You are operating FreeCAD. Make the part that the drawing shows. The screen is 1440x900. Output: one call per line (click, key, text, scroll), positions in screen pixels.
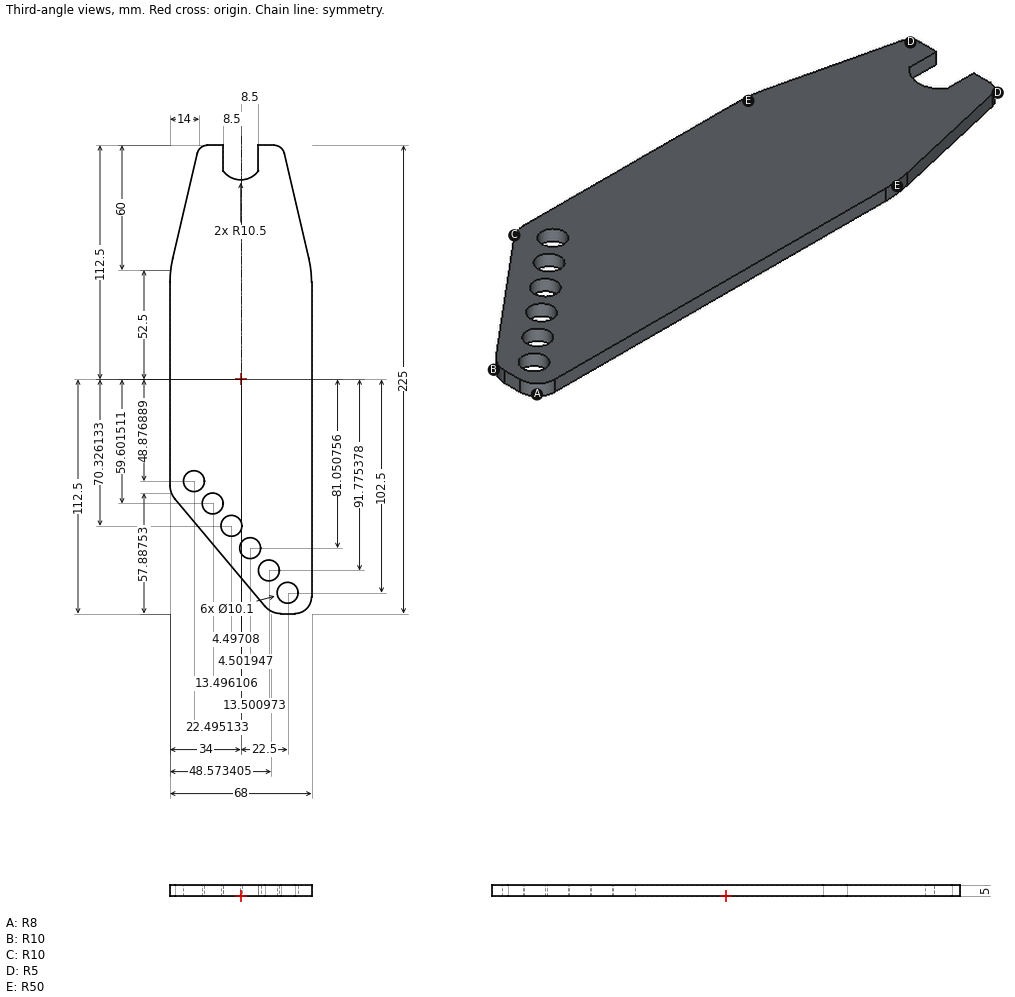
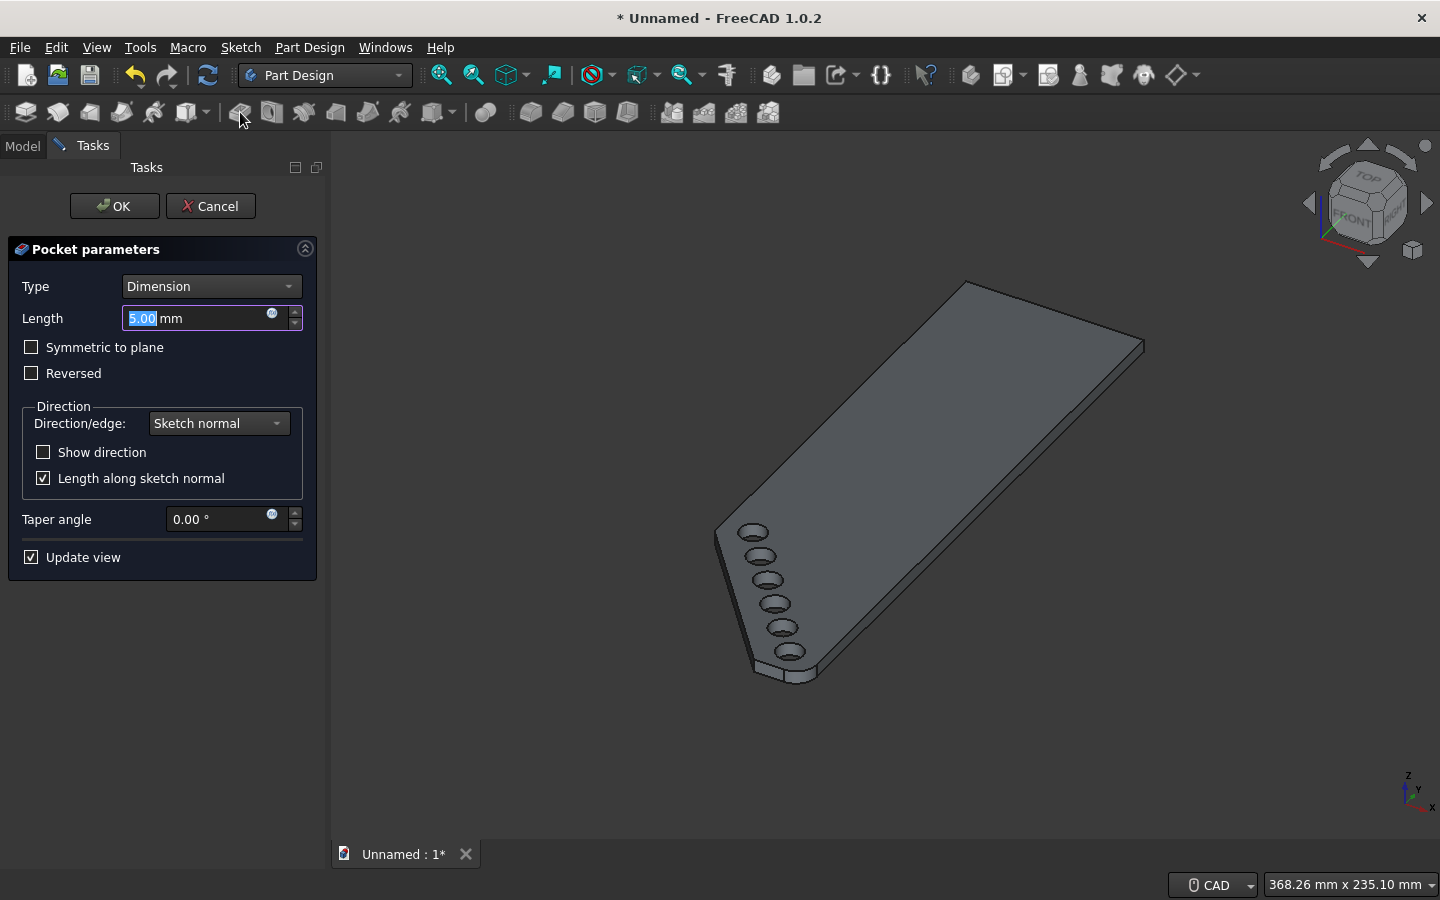
click(212, 286)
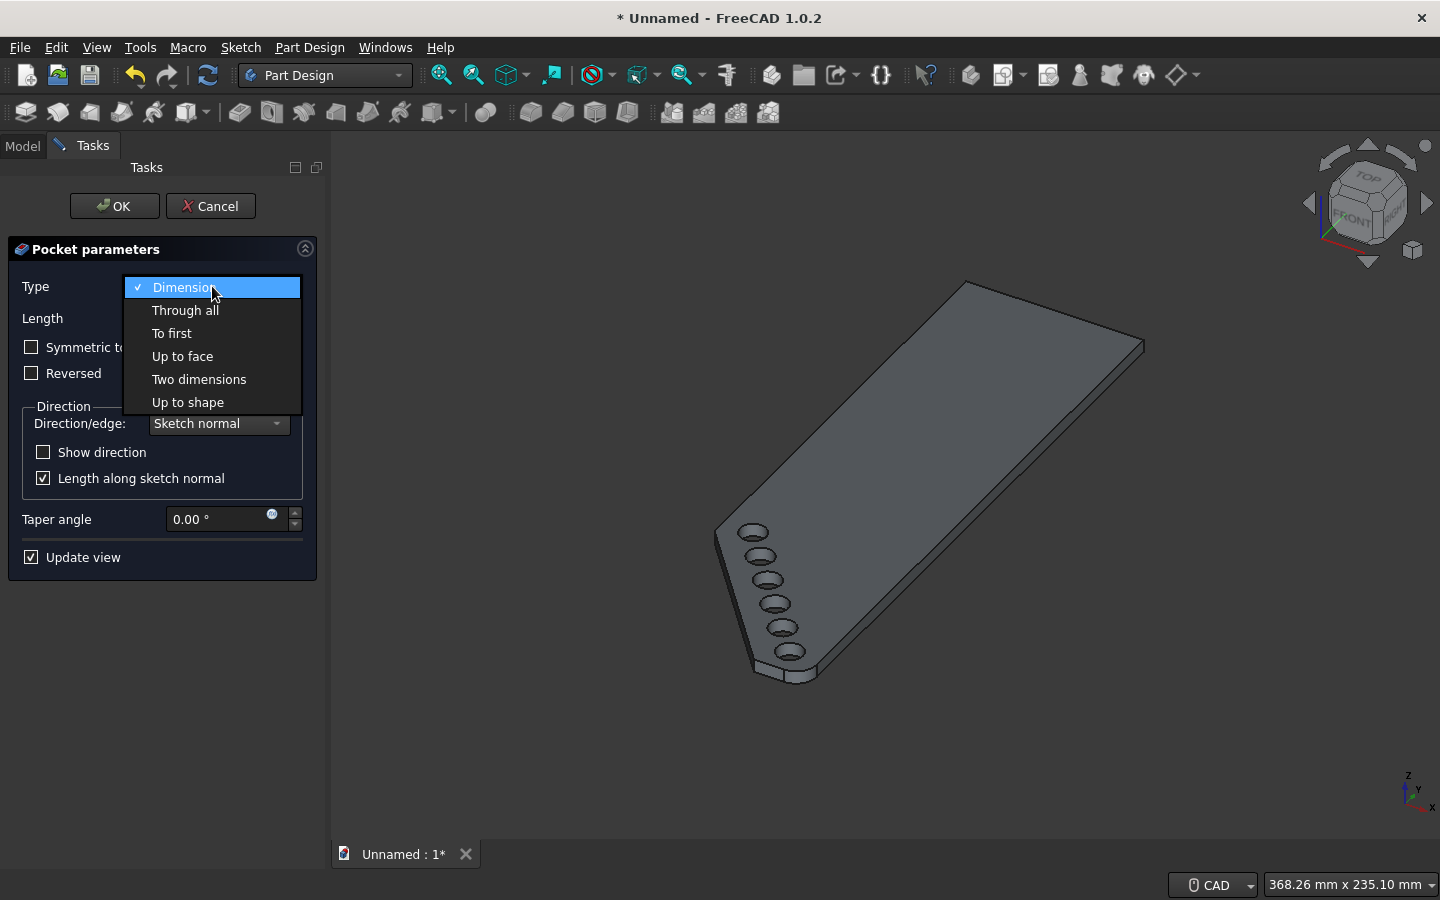
click(212, 310)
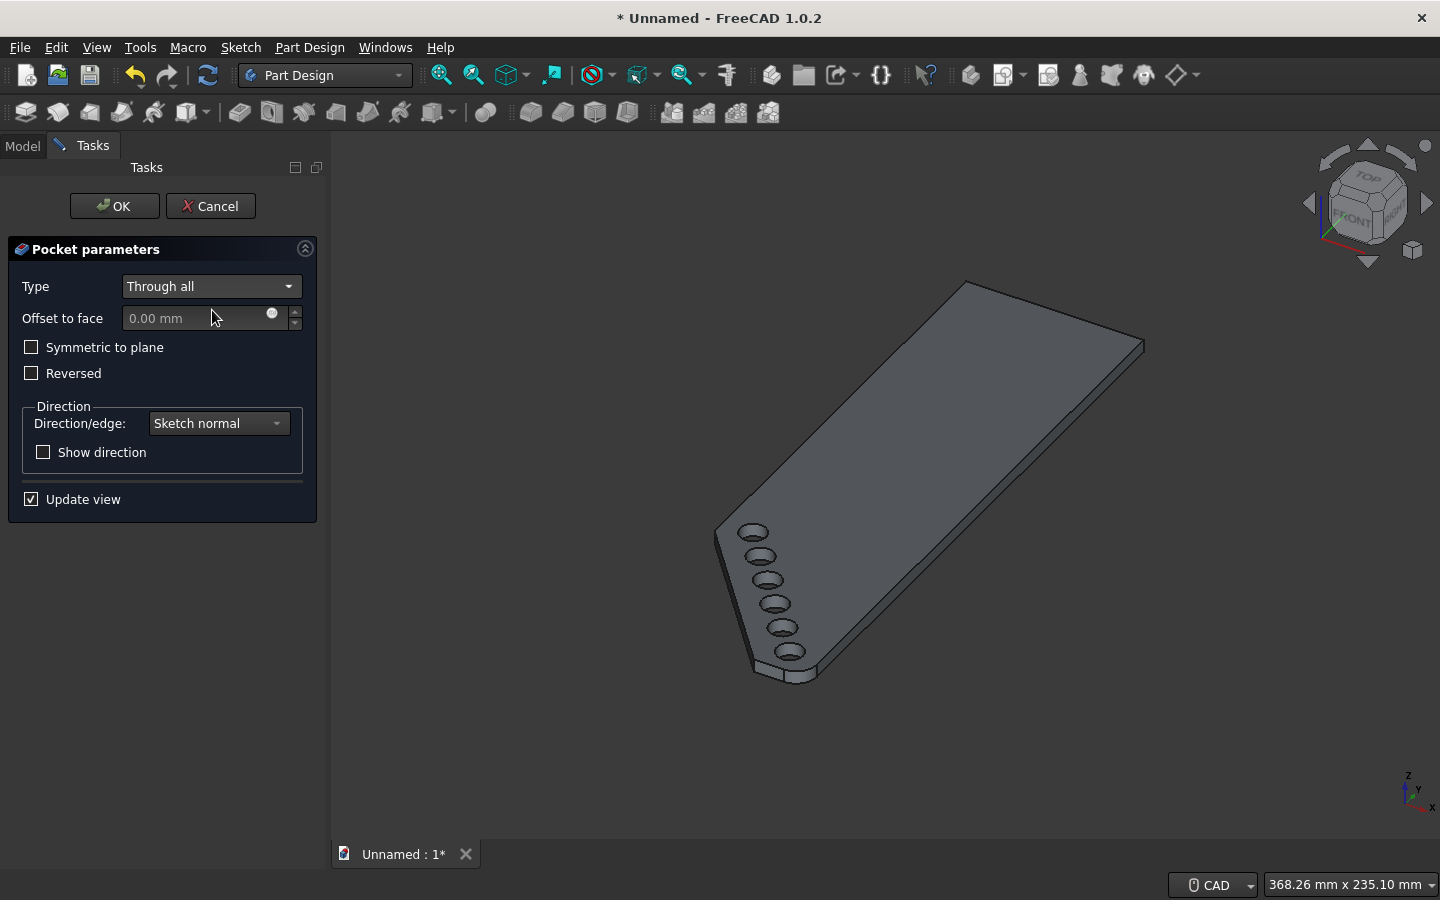
click(115, 206)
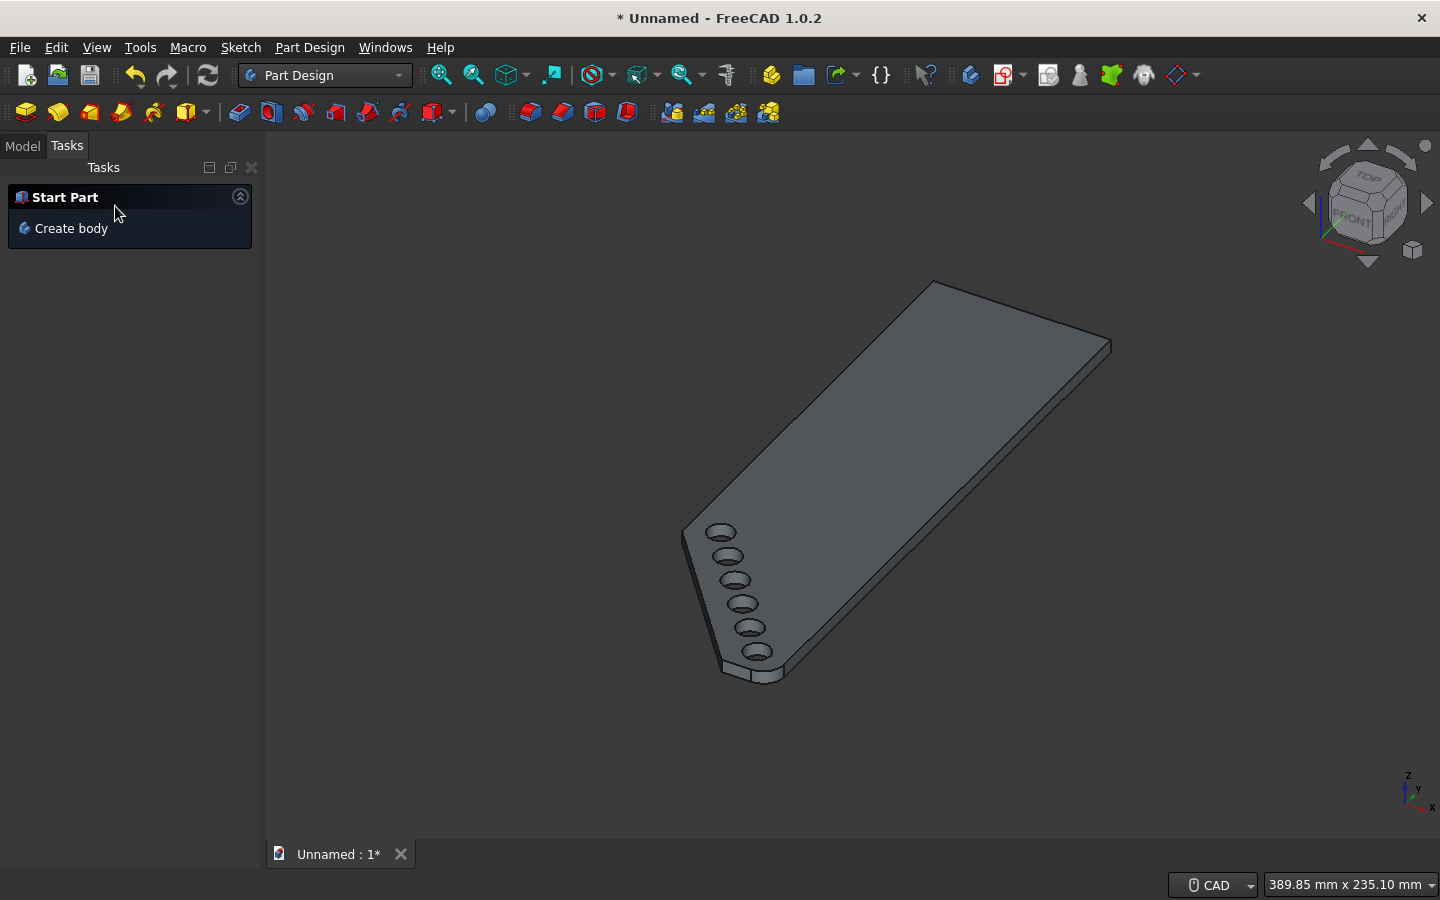
scroll(722, 665, up, 5)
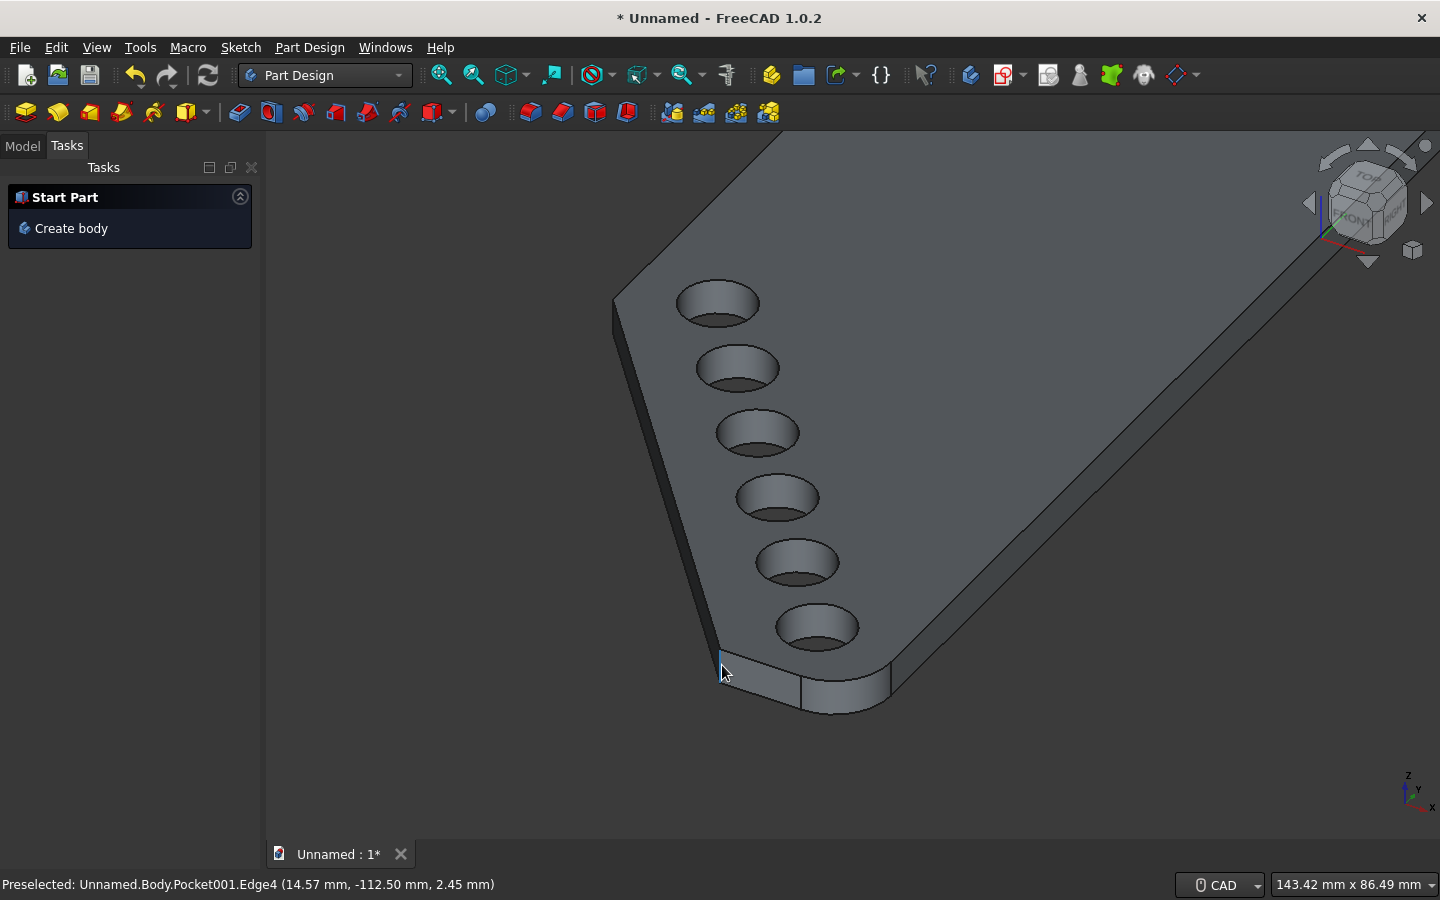
key(v)
key(f)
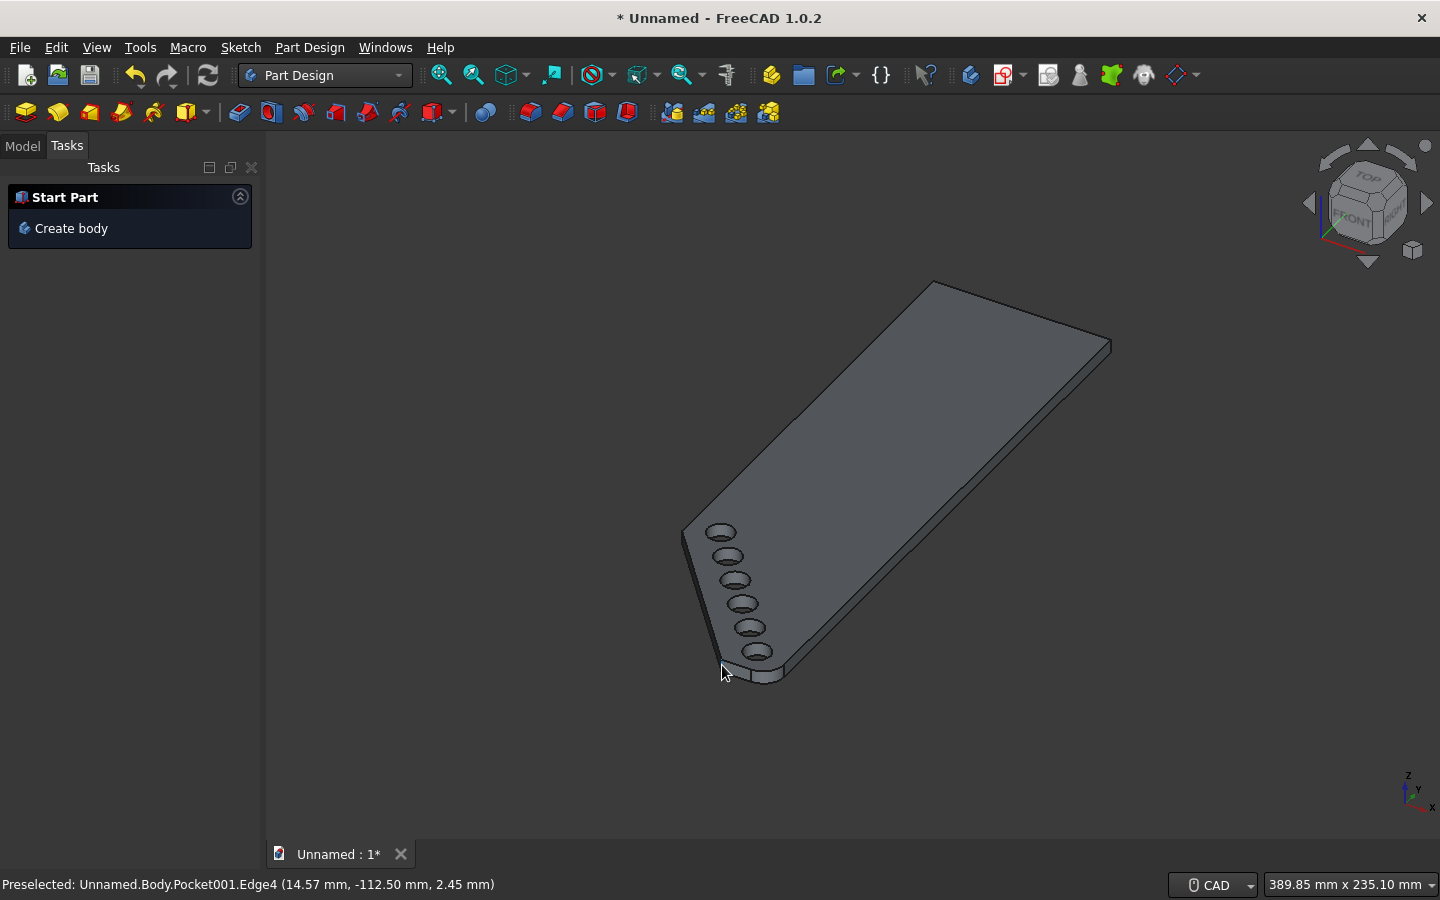
key(0)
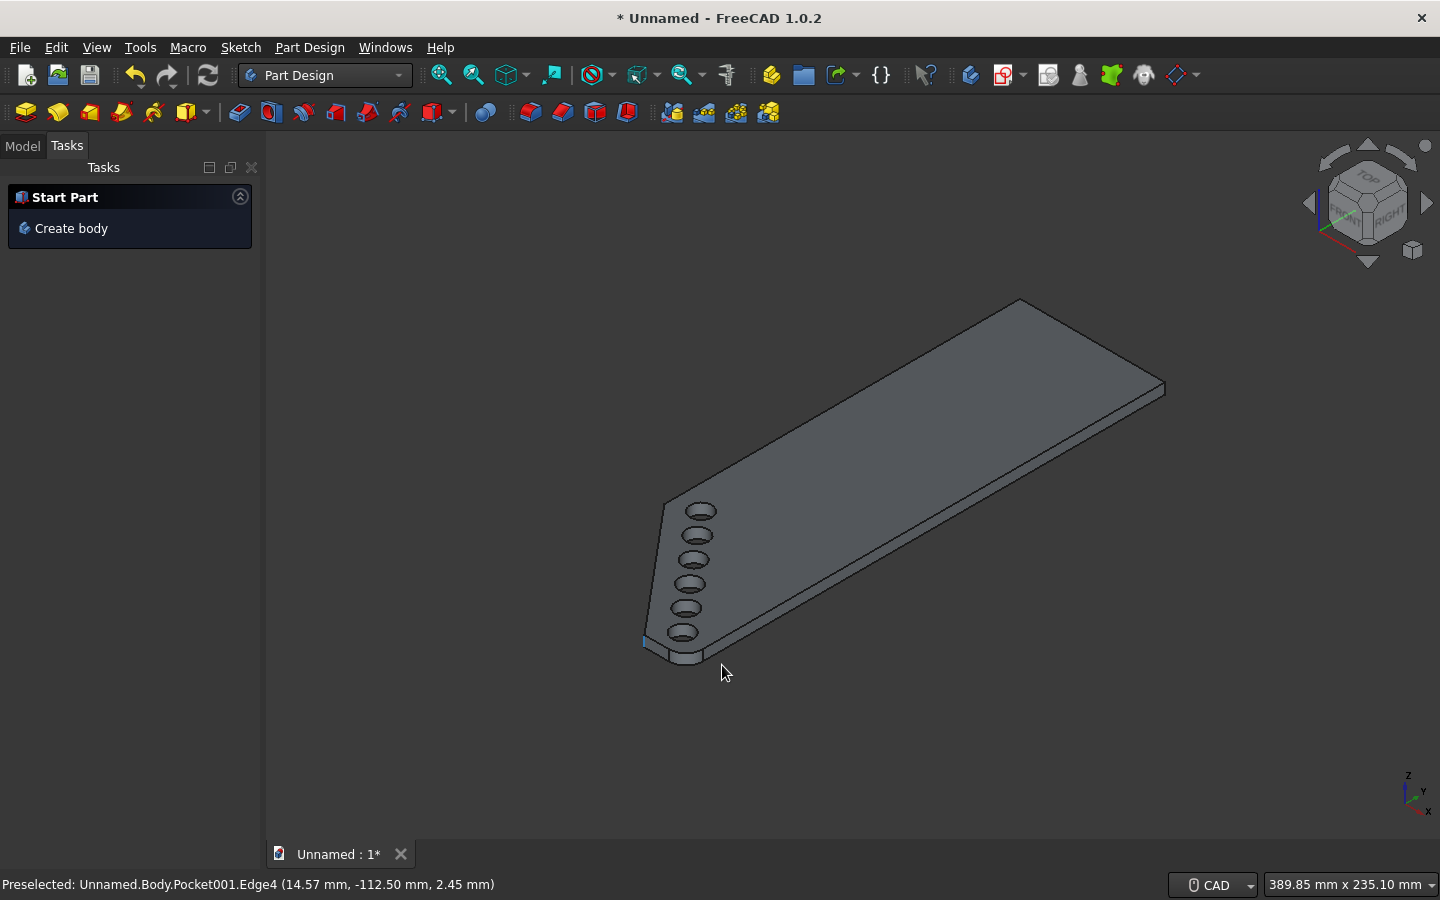
scroll(644, 640, up, 5)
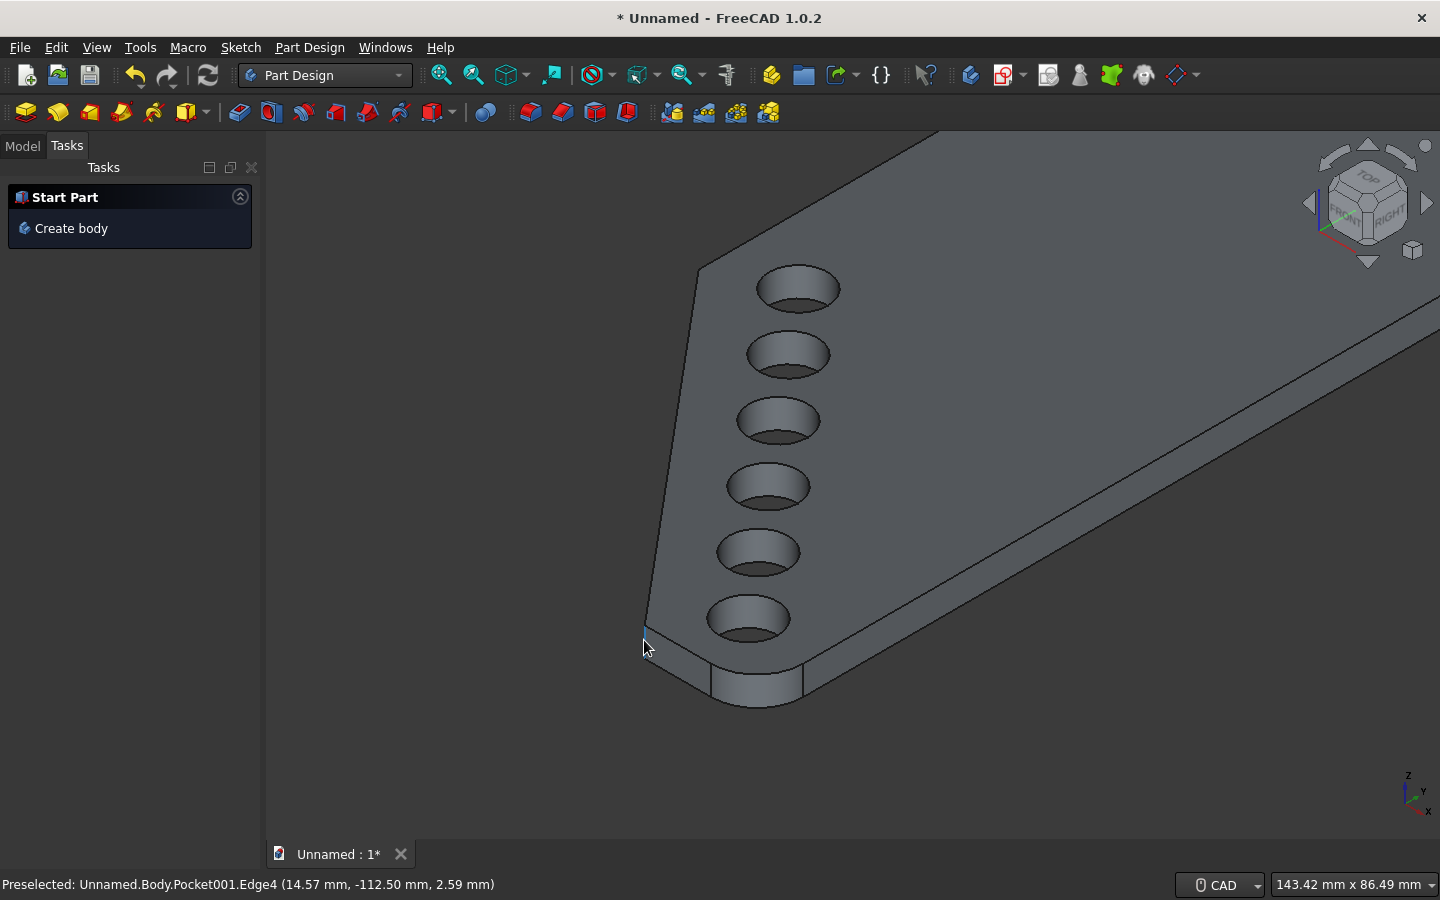
key(v)
key(f)